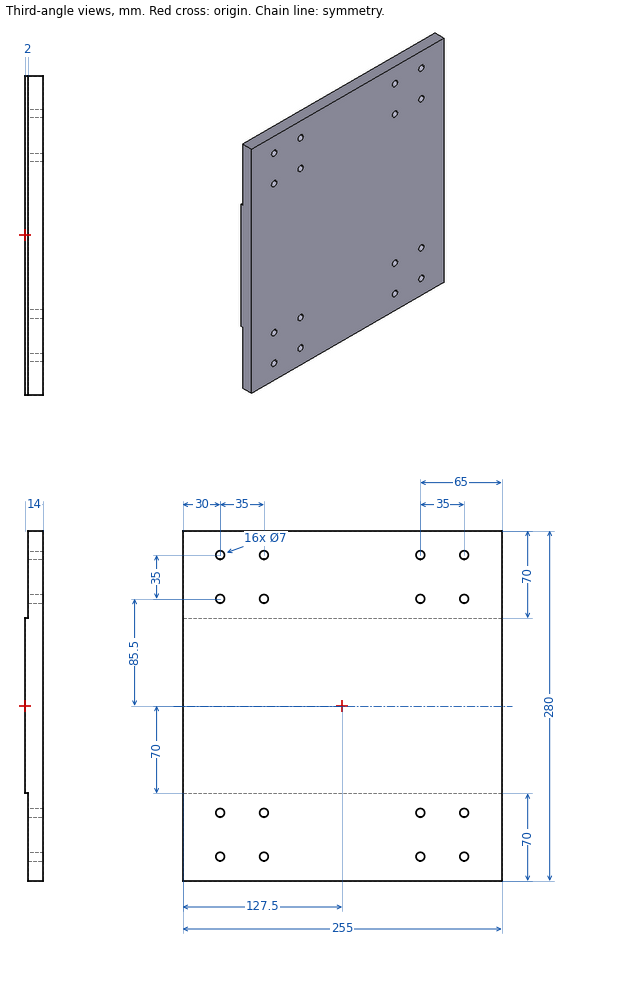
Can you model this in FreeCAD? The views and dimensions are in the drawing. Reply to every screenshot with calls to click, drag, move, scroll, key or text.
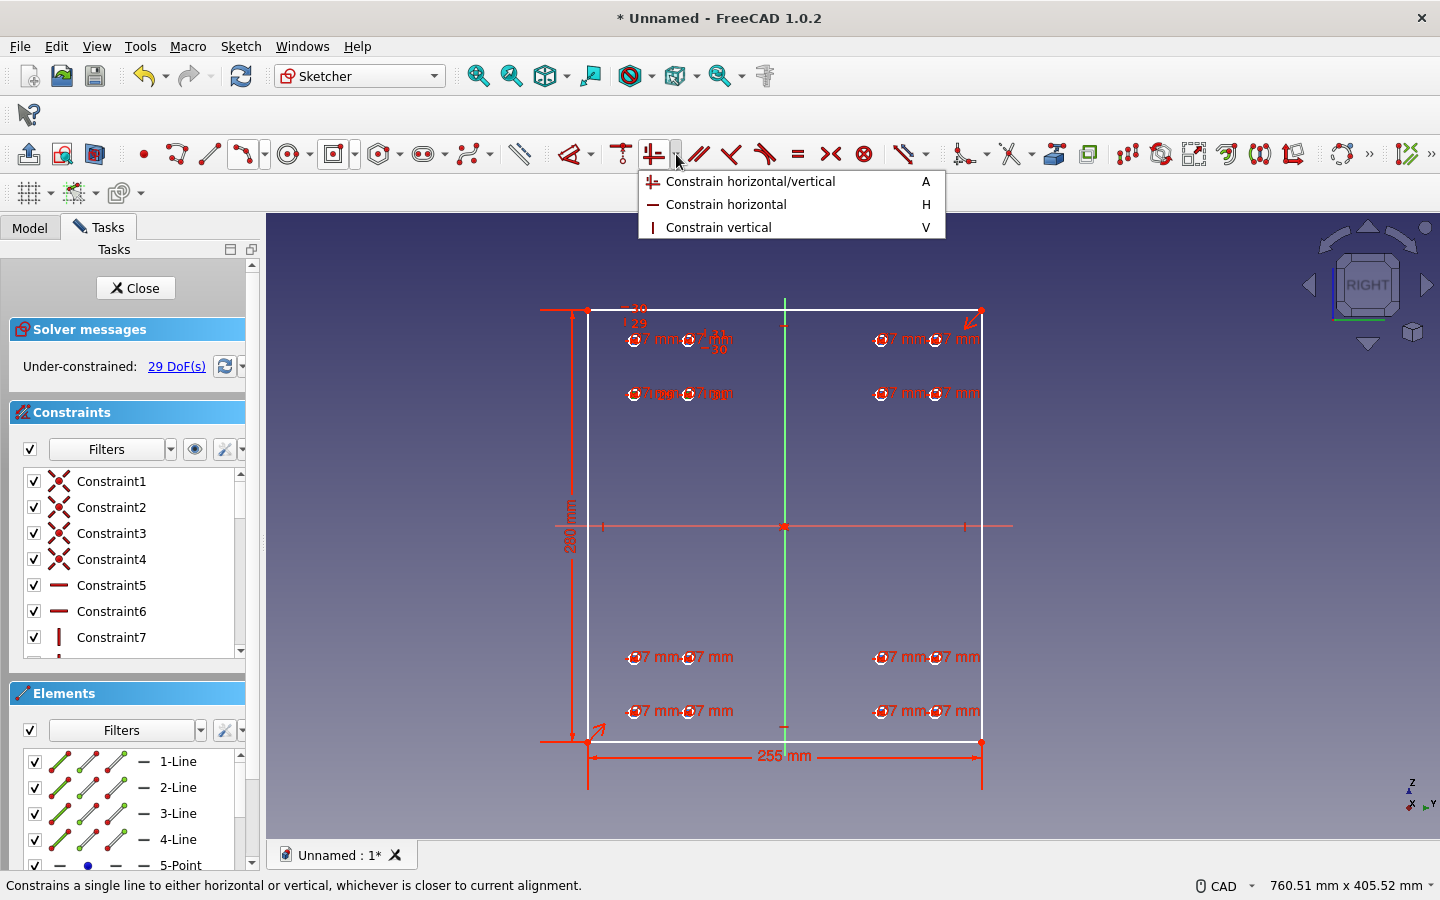
click(792, 204)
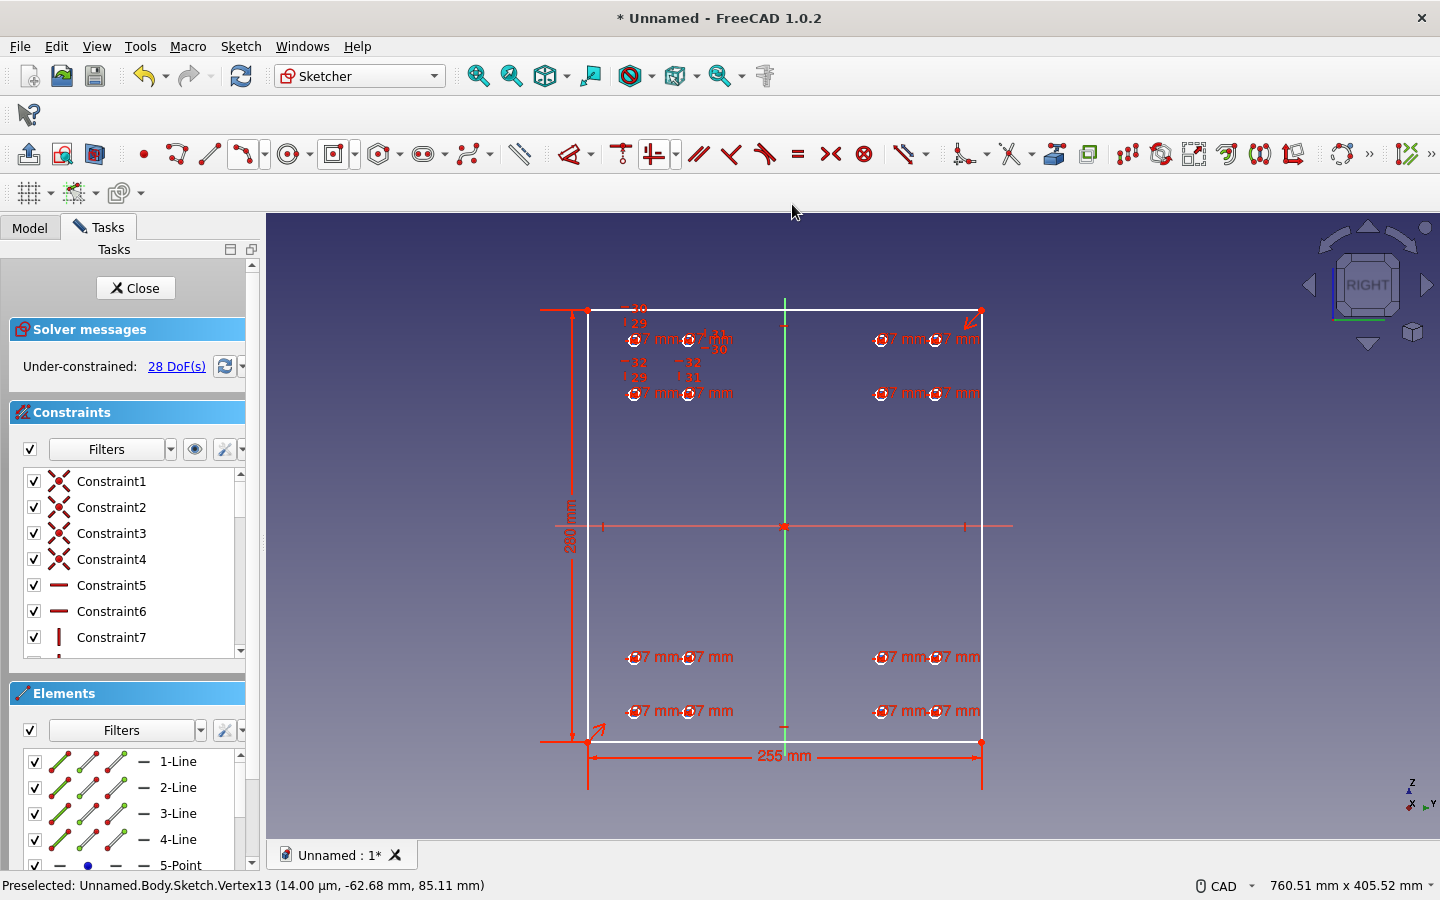
click(634, 395)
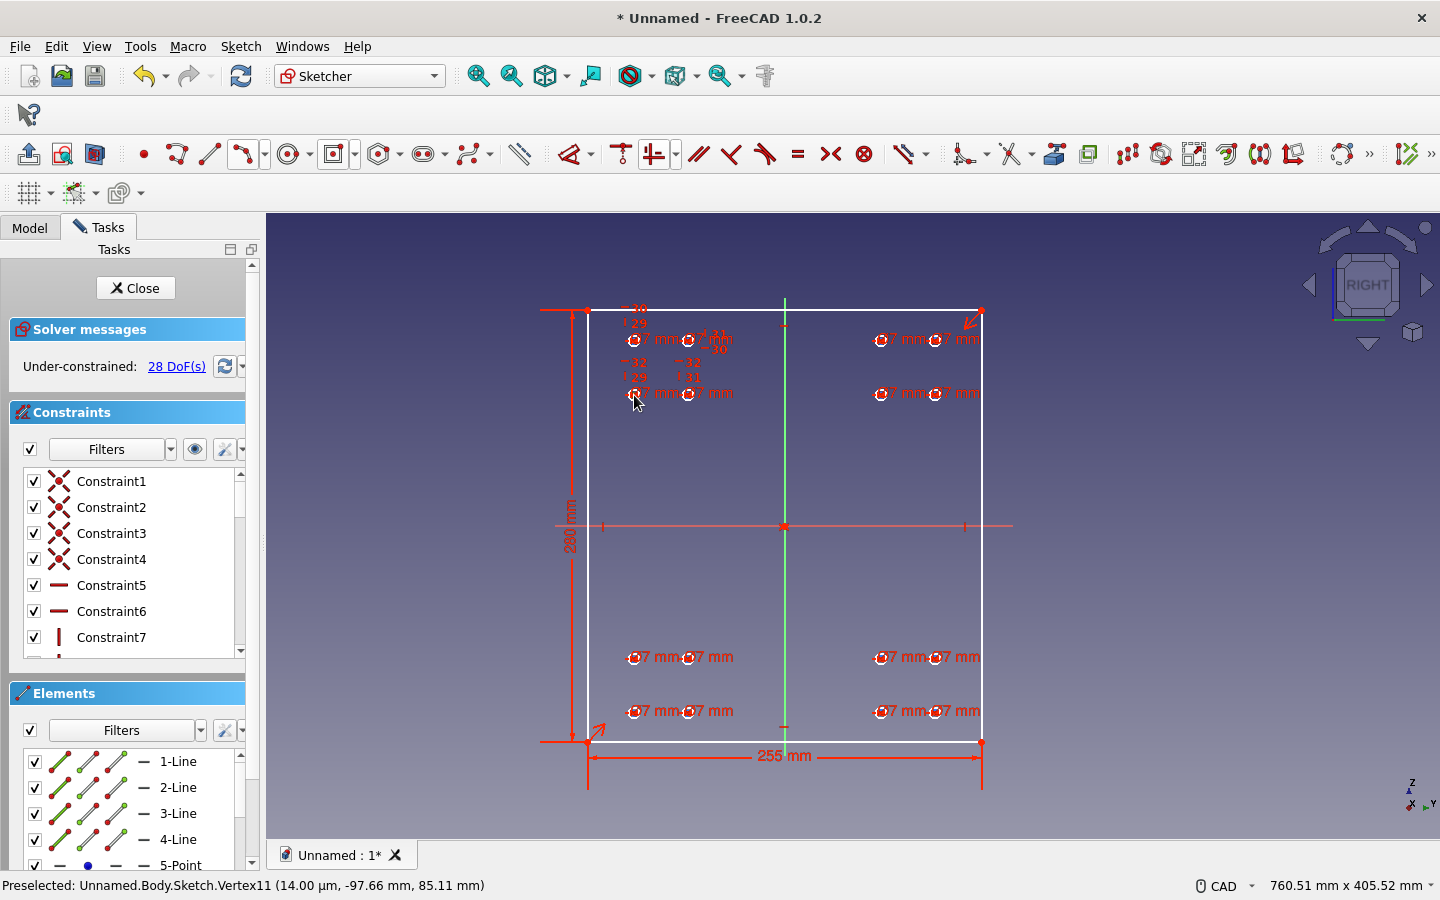
click(634, 659)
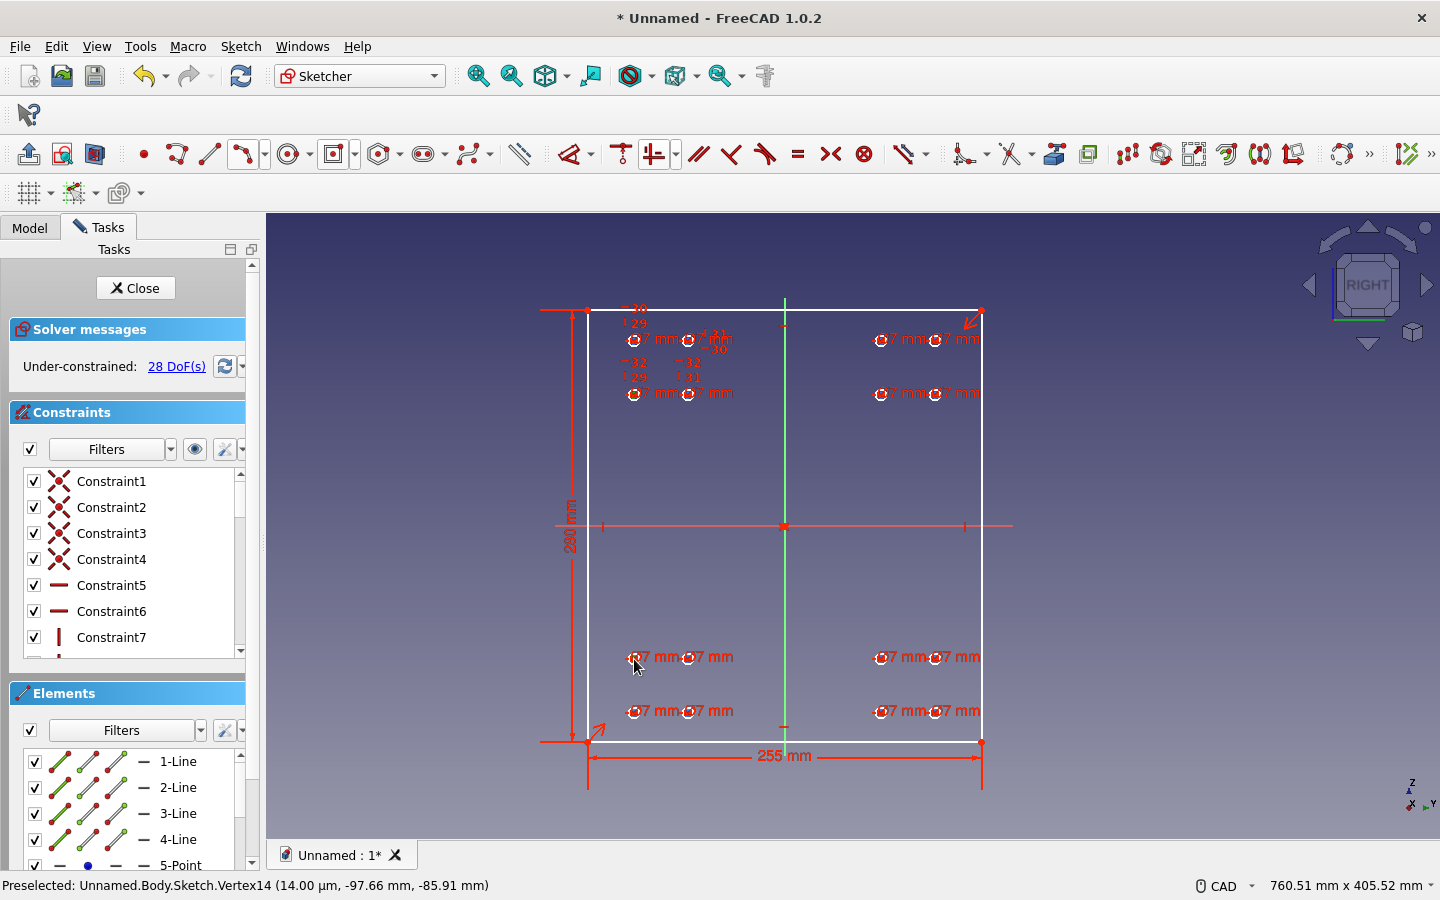
click(676, 154)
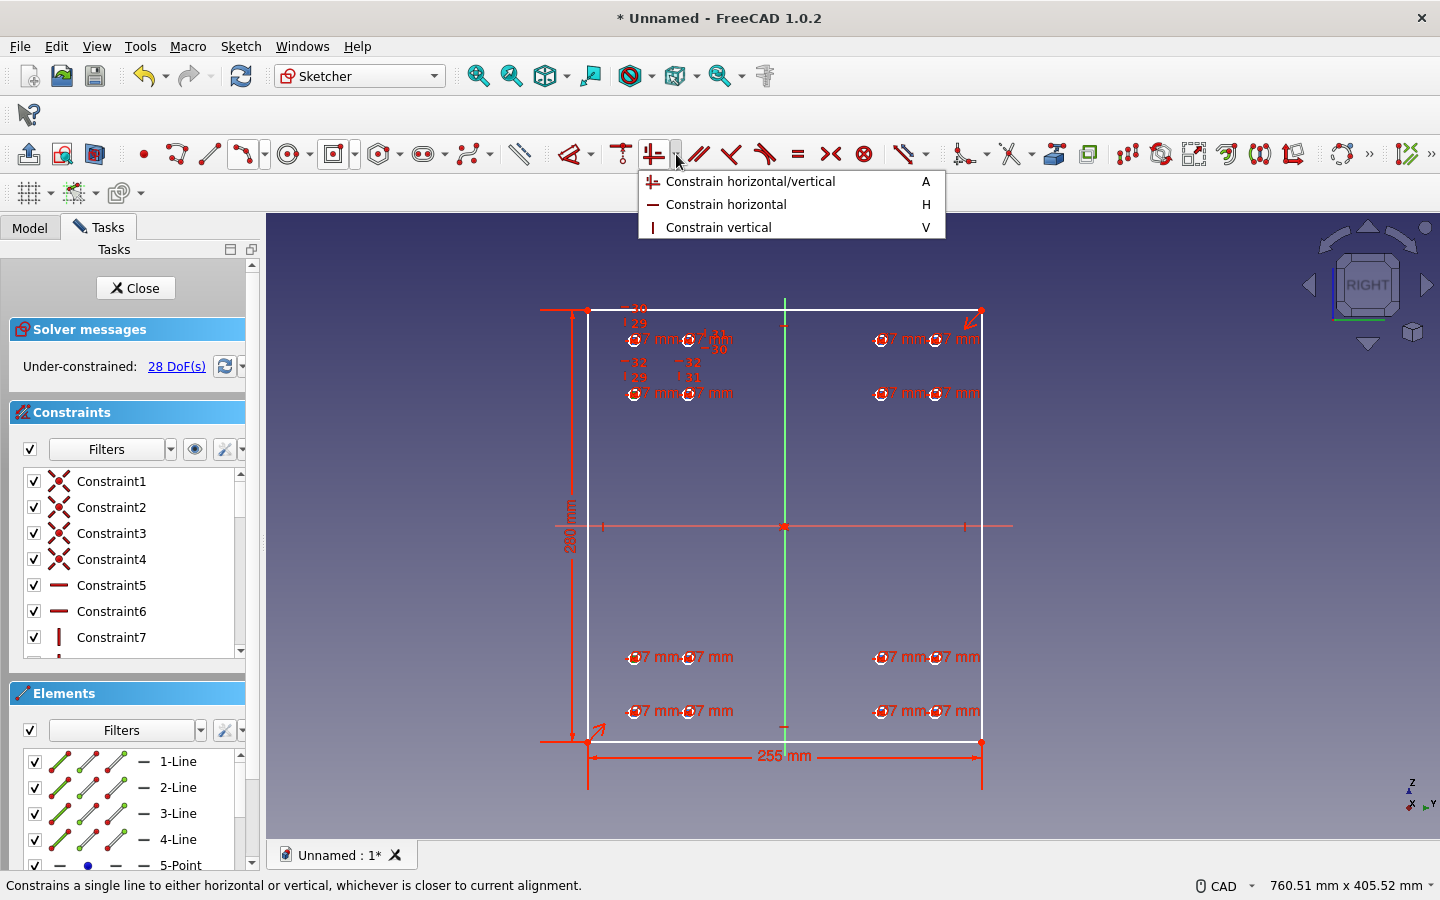
click(792, 228)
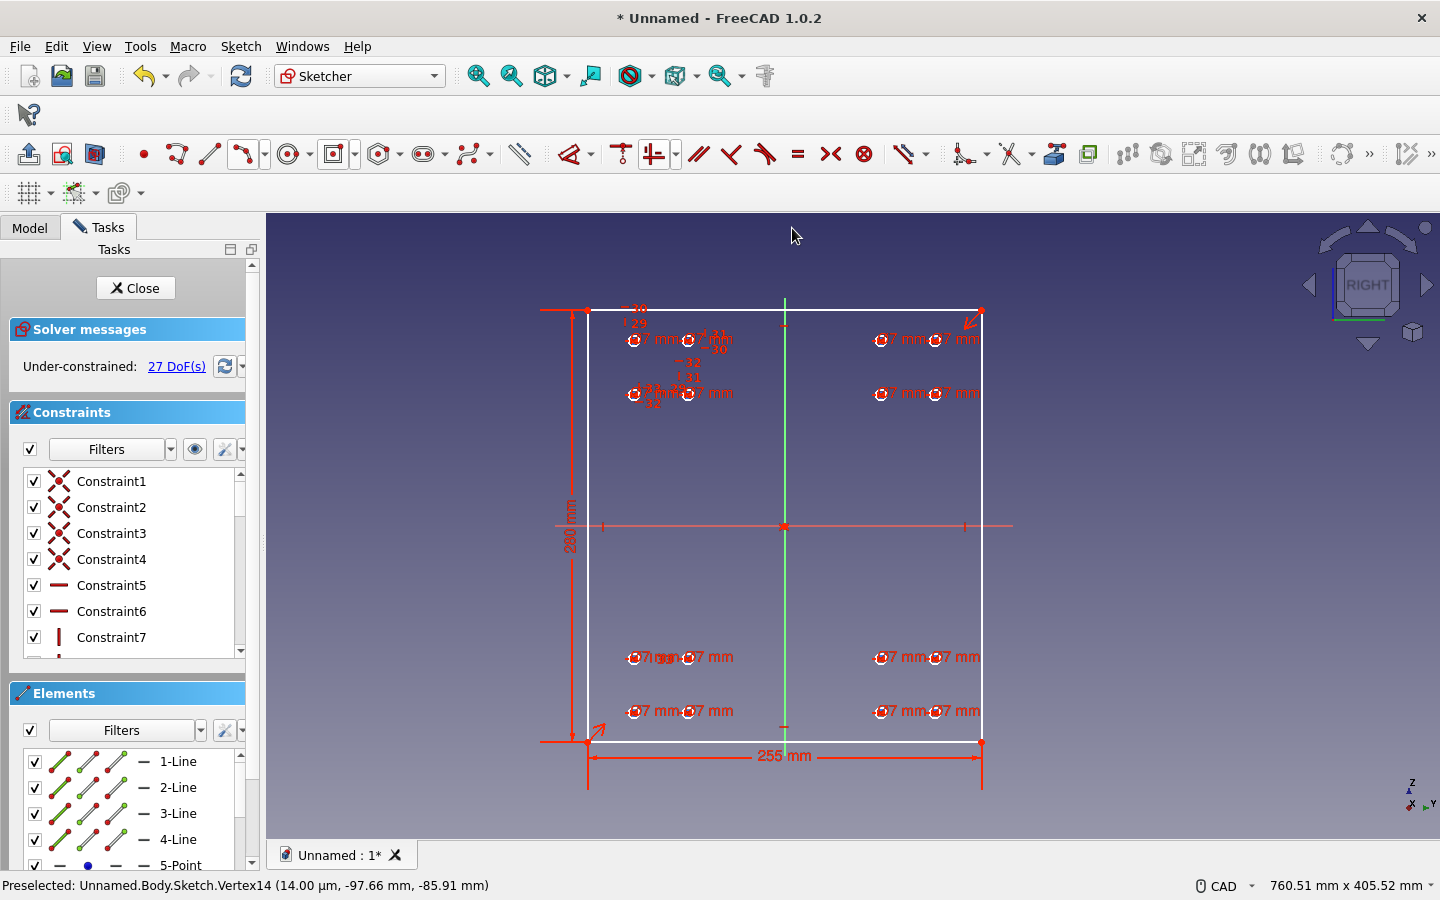
click(634, 659)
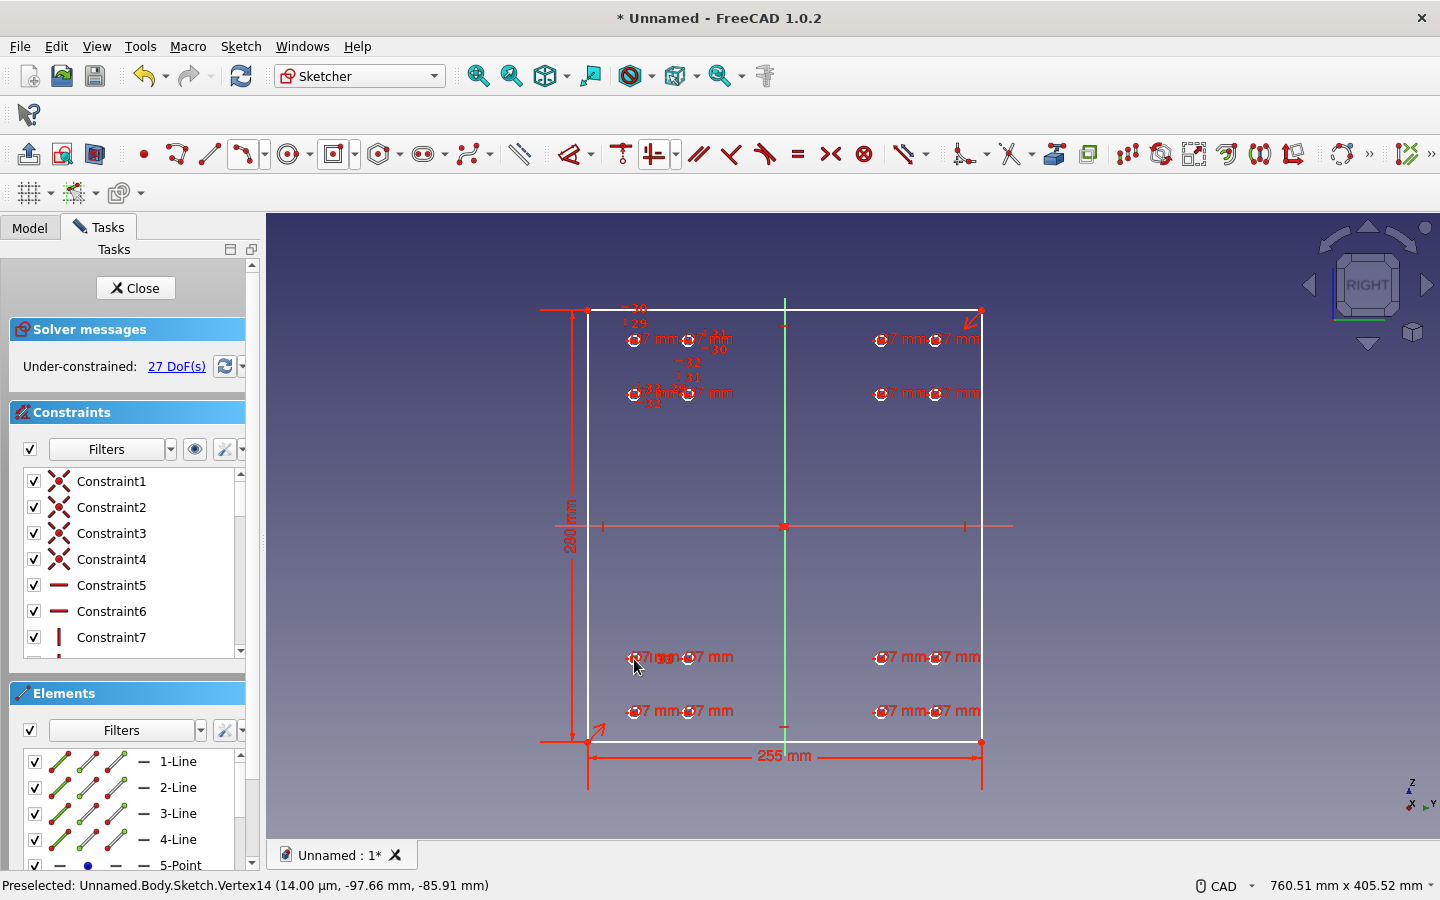
click(634, 713)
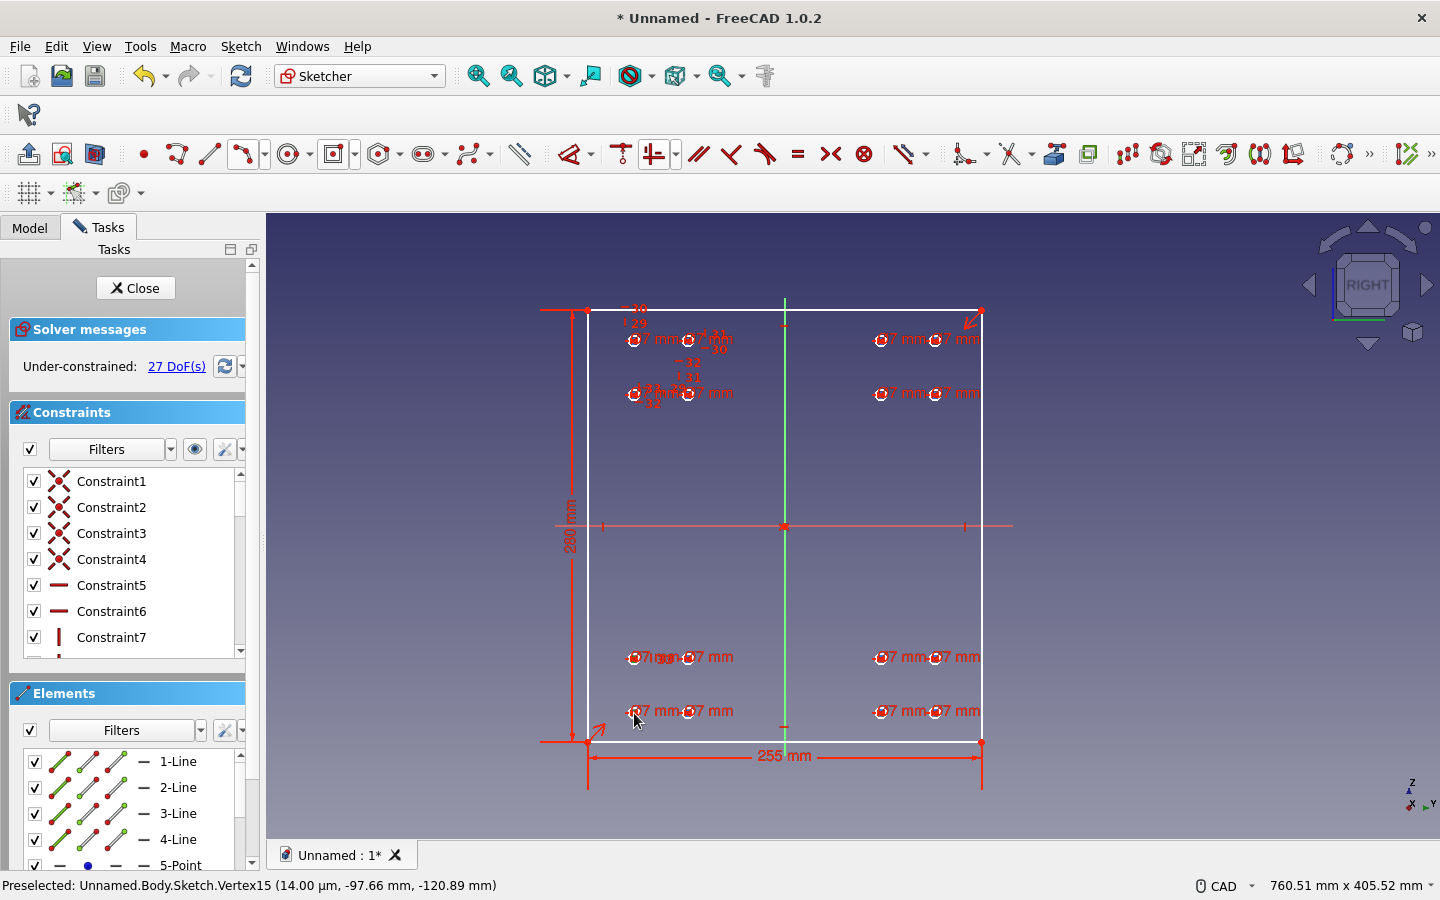
click(676, 154)